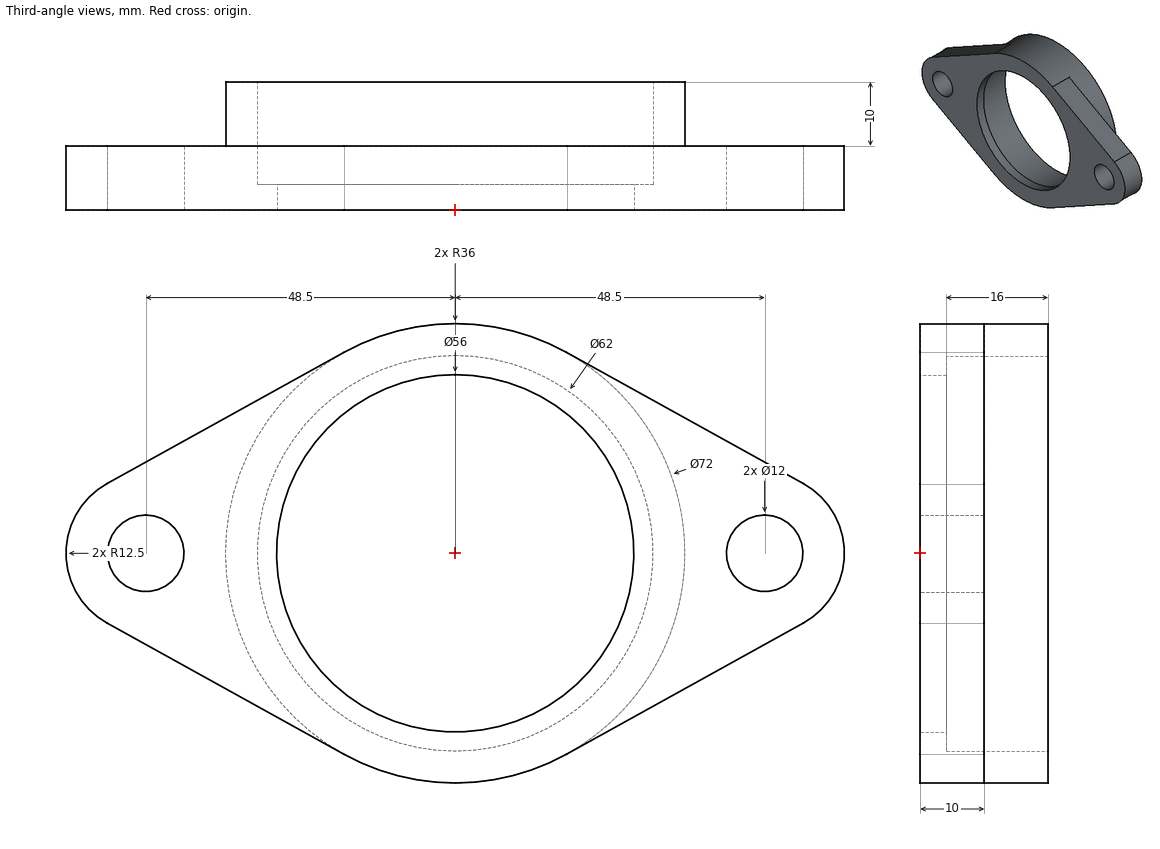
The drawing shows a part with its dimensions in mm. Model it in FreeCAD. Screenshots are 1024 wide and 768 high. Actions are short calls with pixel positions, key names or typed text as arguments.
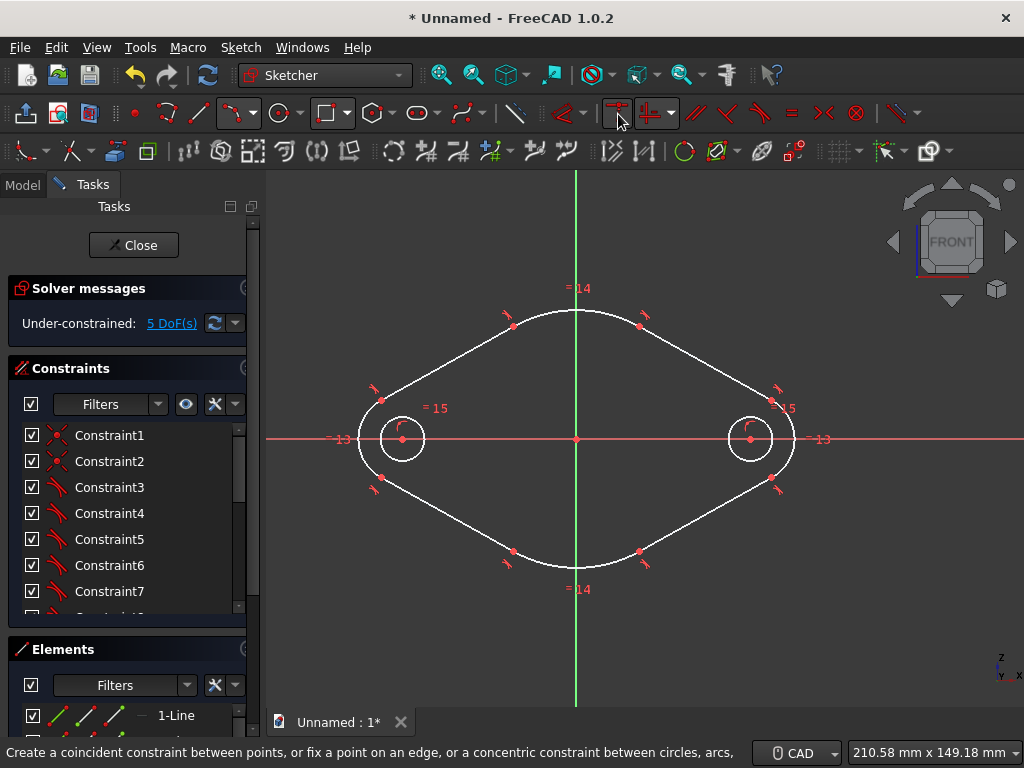
click(362, 421)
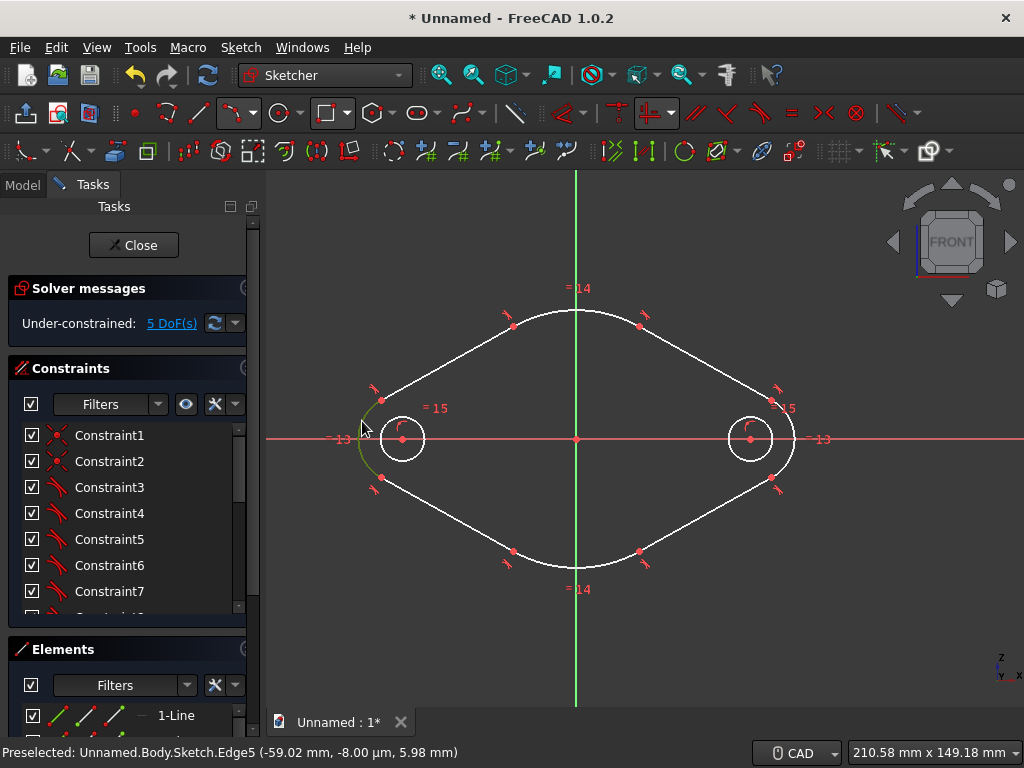
click(586, 114)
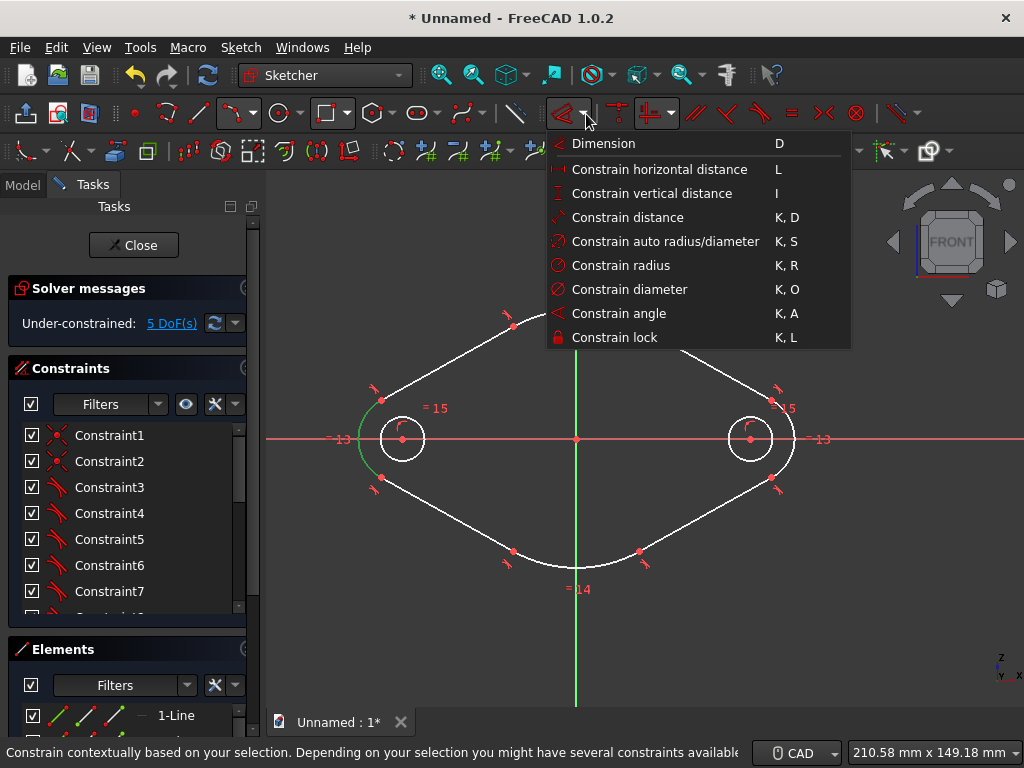
click(699, 265)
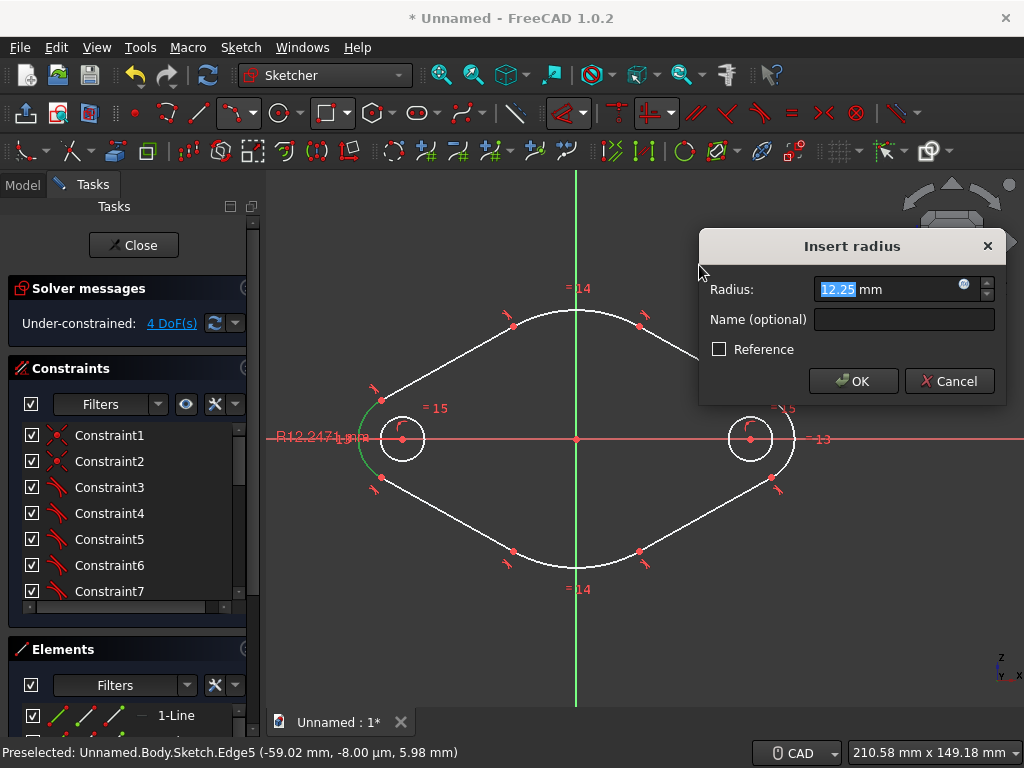
text(12.5)
key(Return)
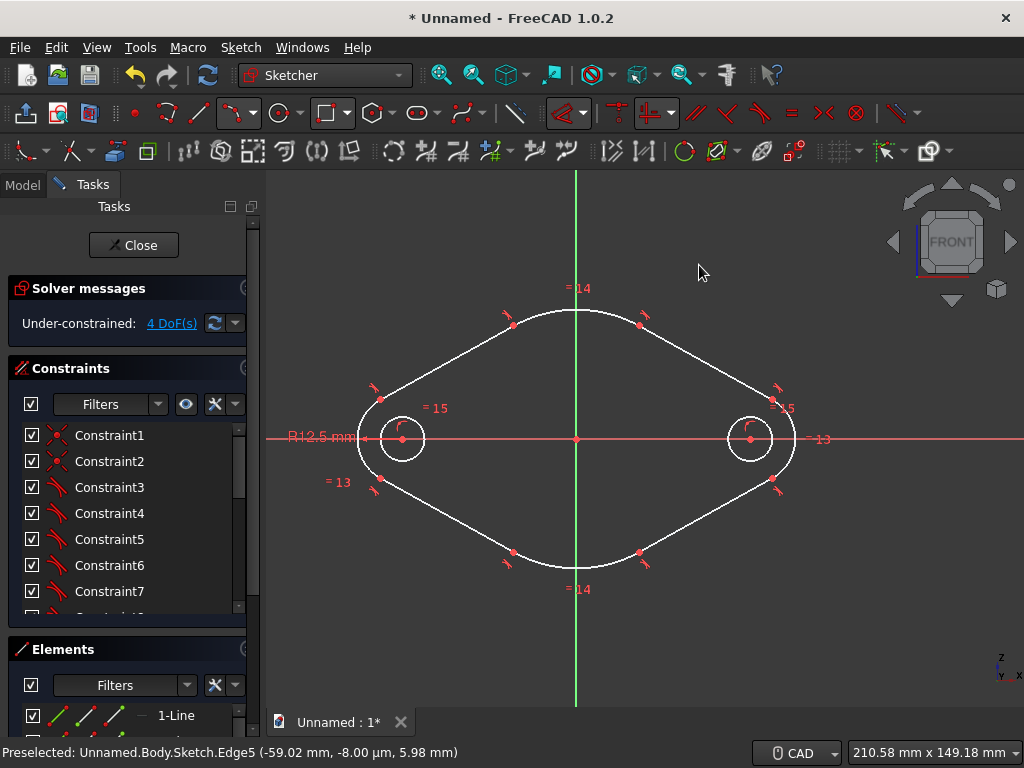
click(603, 312)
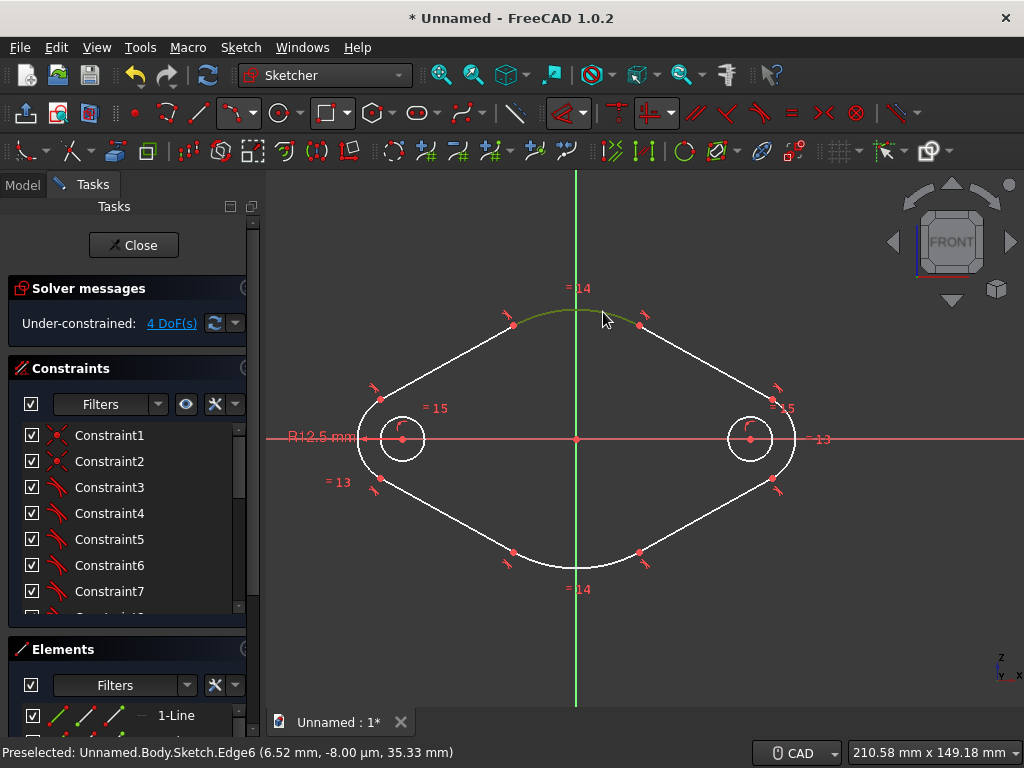
click(586, 114)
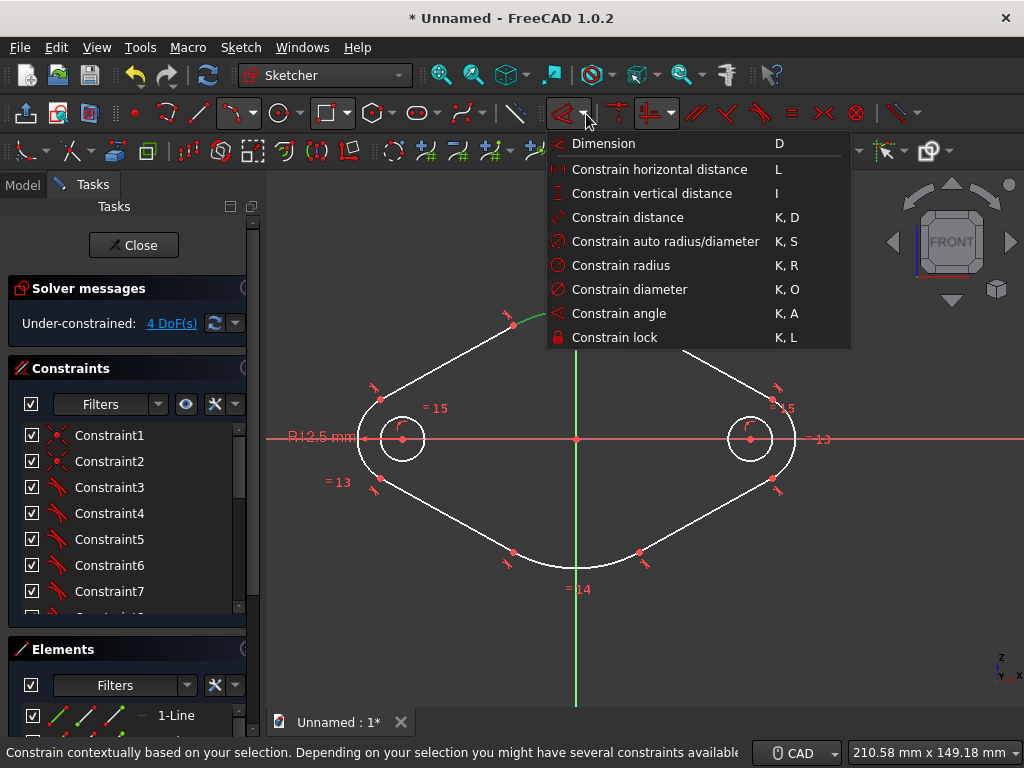
click(699, 265)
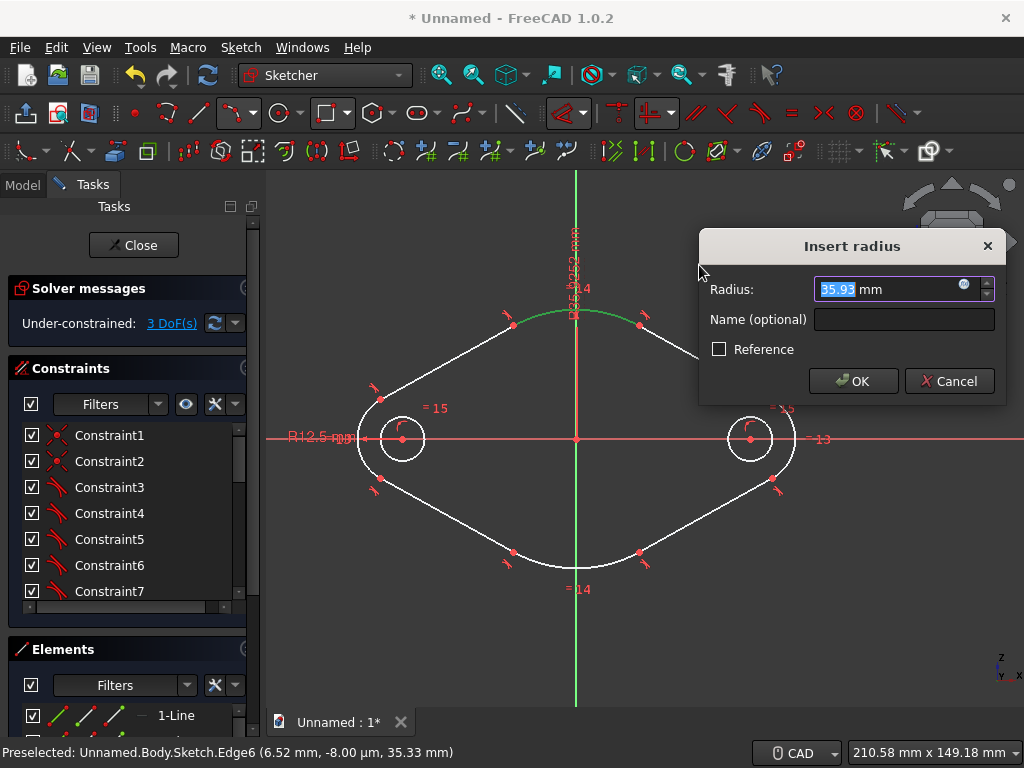
text(36)
key(Return)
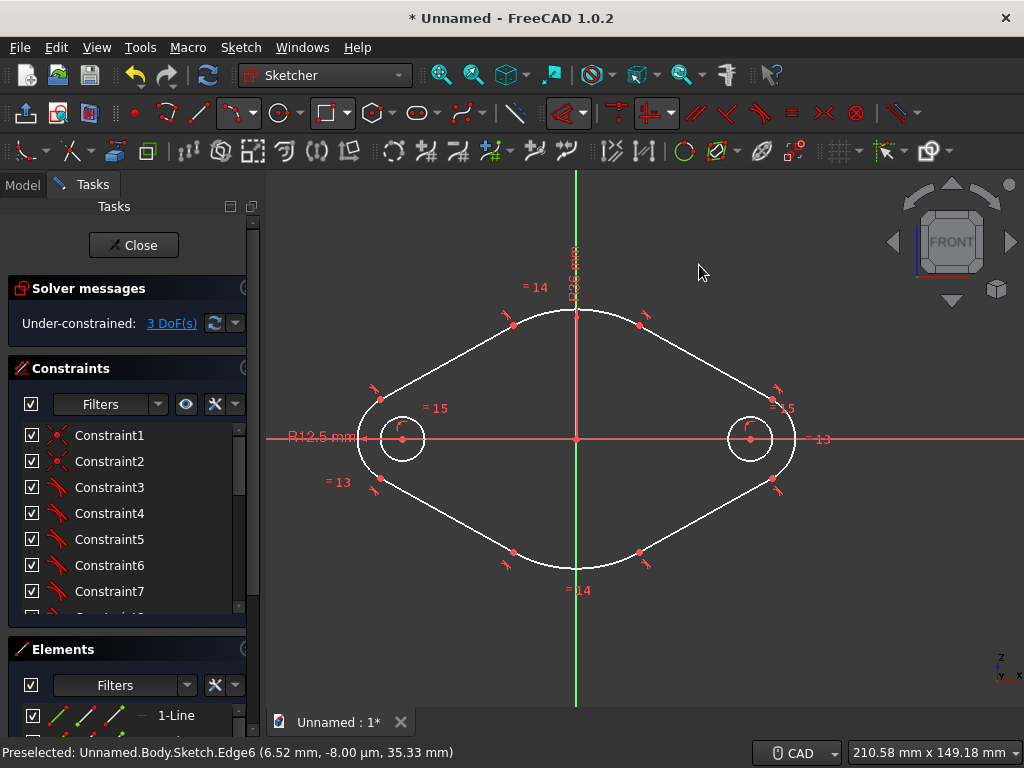
click(766, 423)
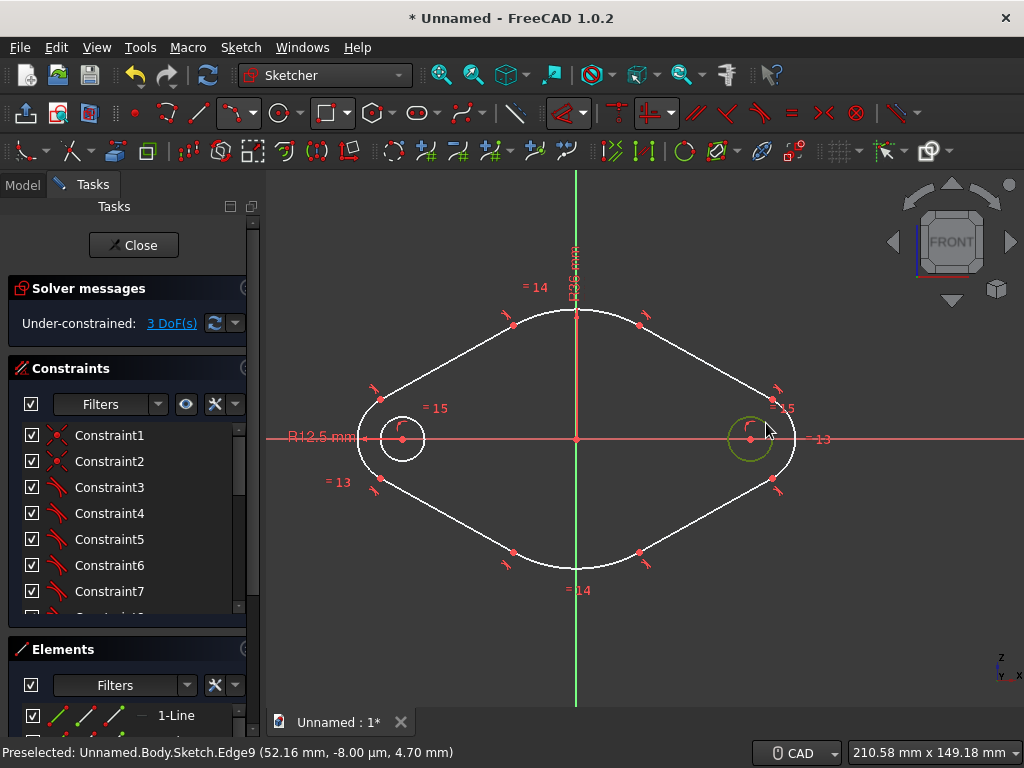
click(586, 114)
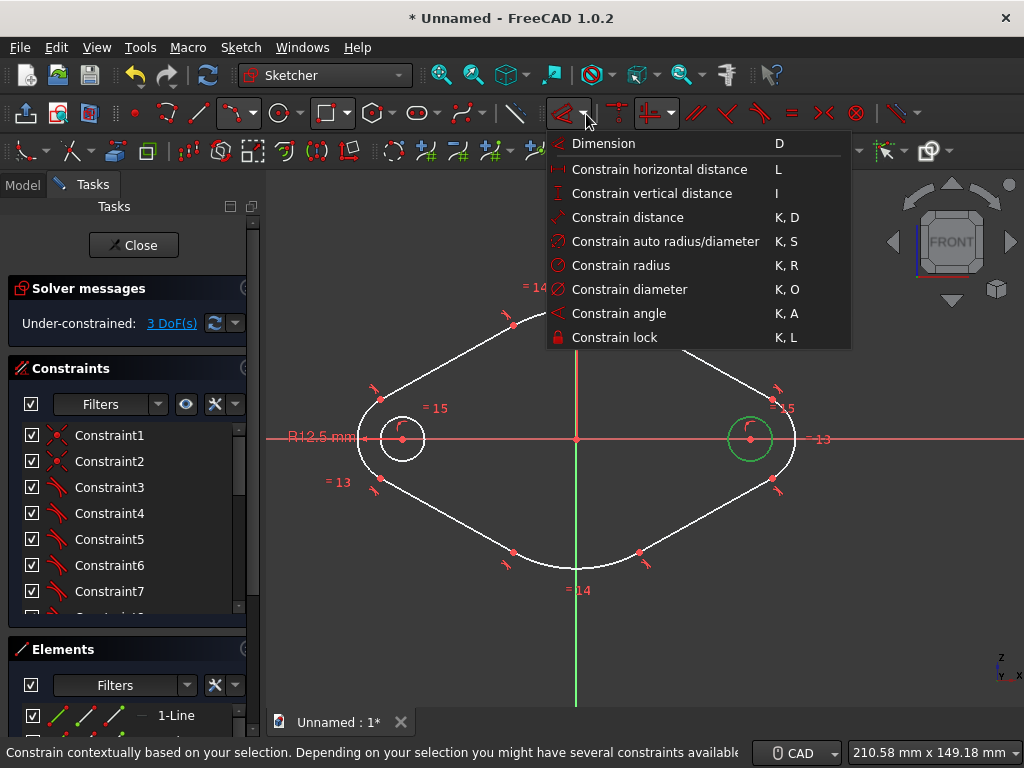
click(699, 289)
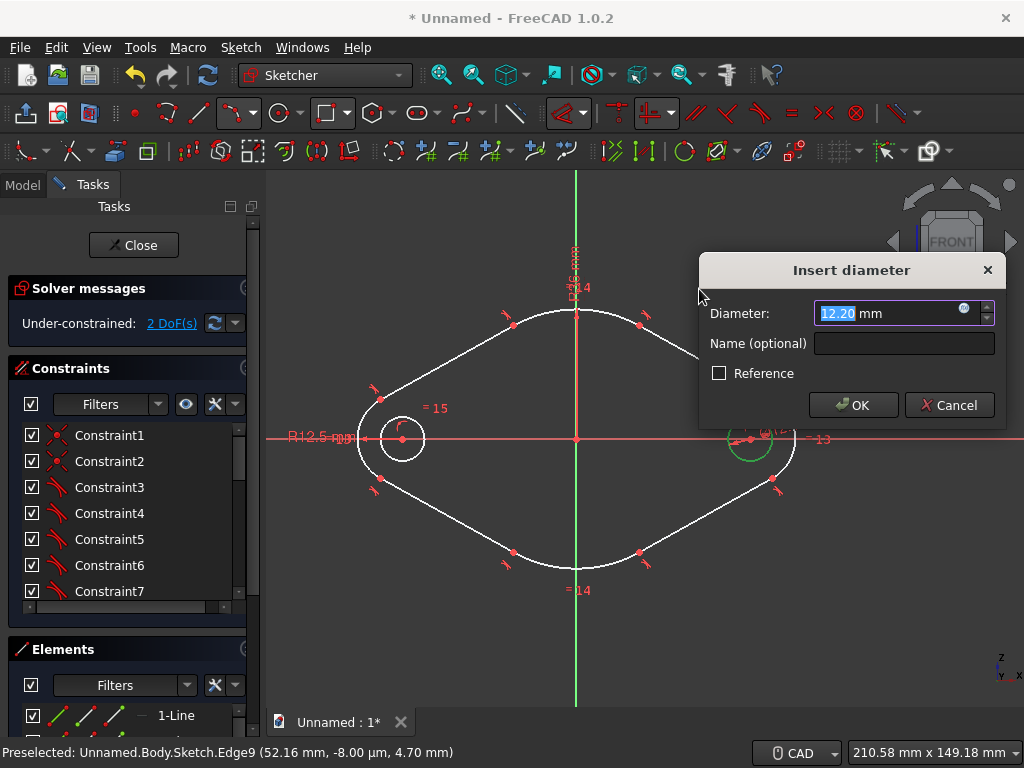
text(12)
key(Return)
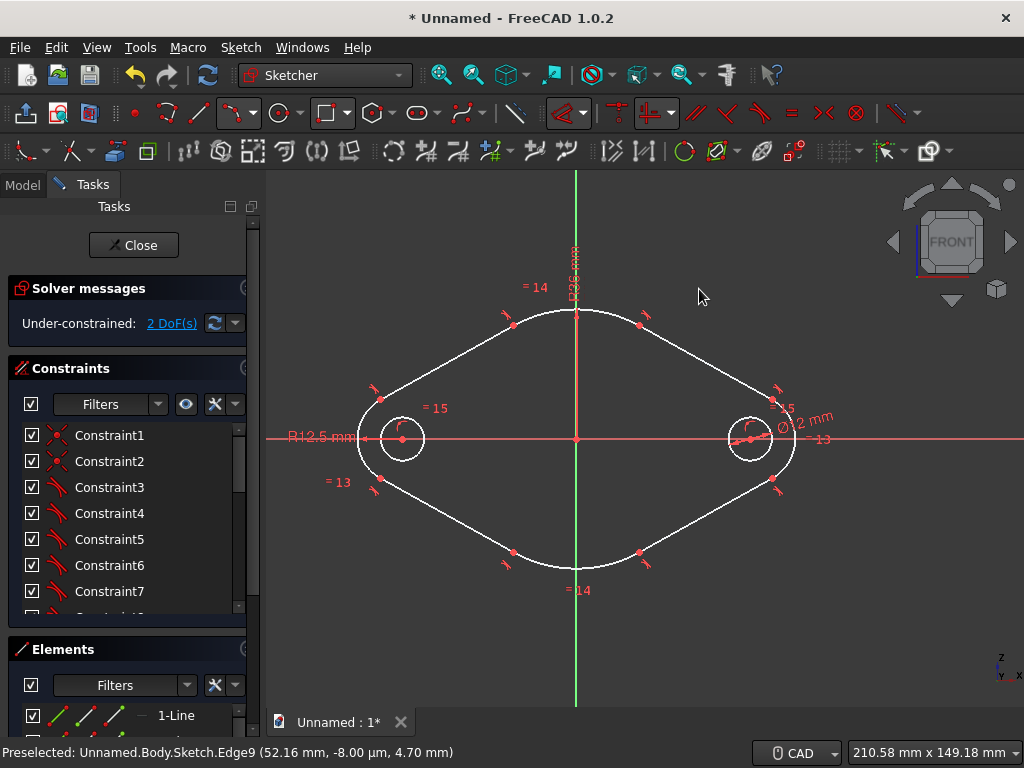
click(750, 439)